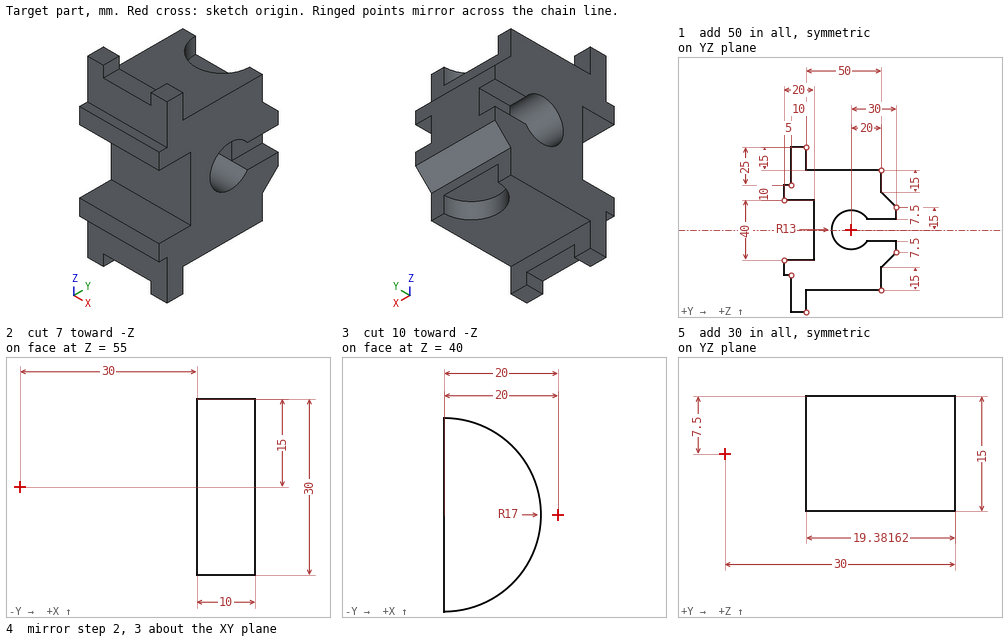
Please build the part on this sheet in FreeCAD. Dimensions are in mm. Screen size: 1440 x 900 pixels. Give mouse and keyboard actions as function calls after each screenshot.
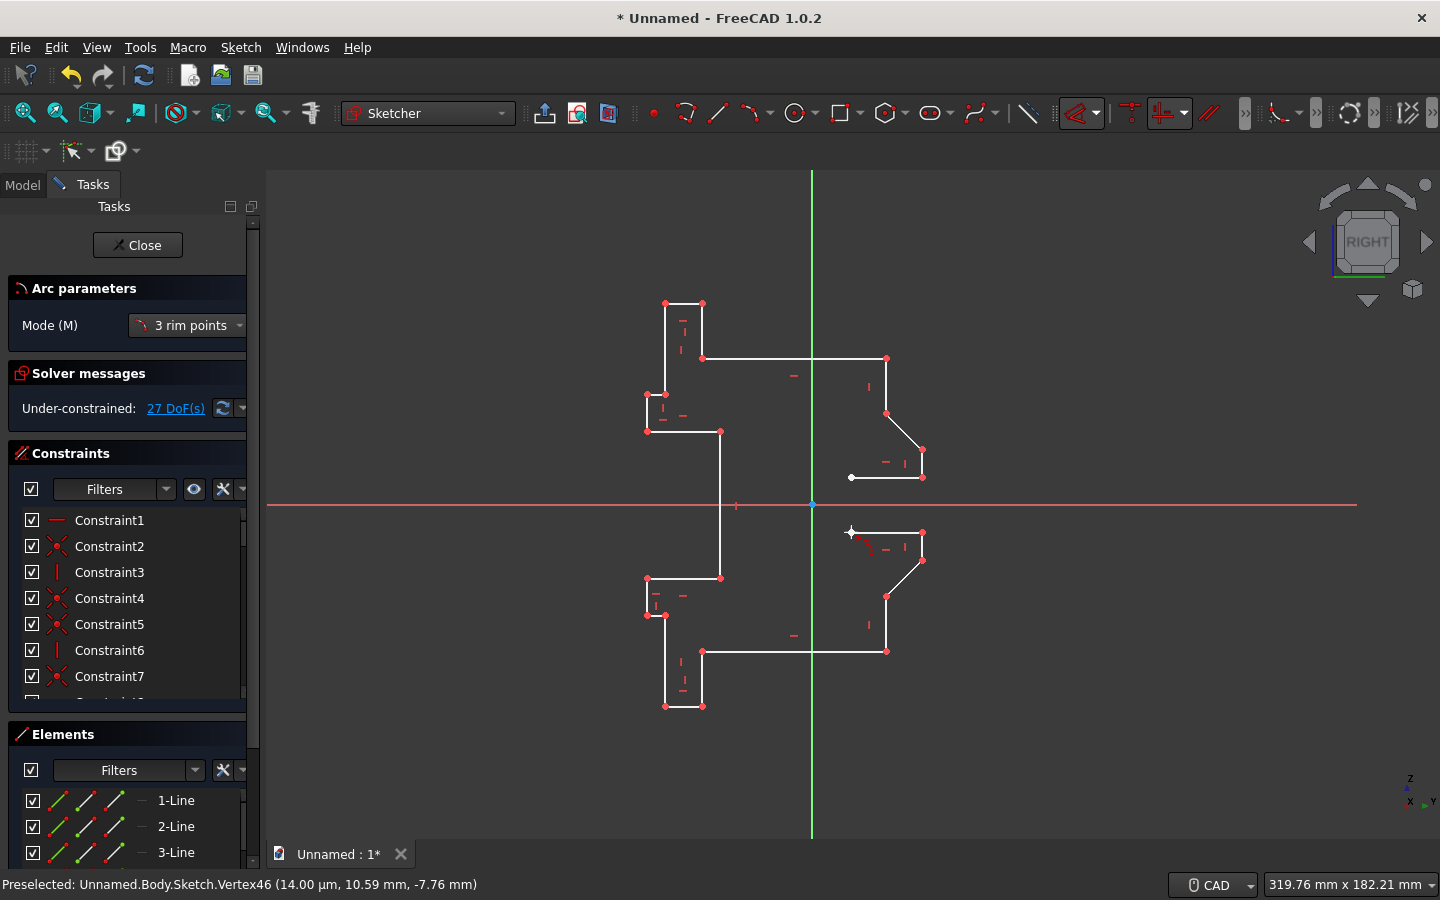
click(851, 533)
click(851, 478)
click(770, 481)
key(Escape)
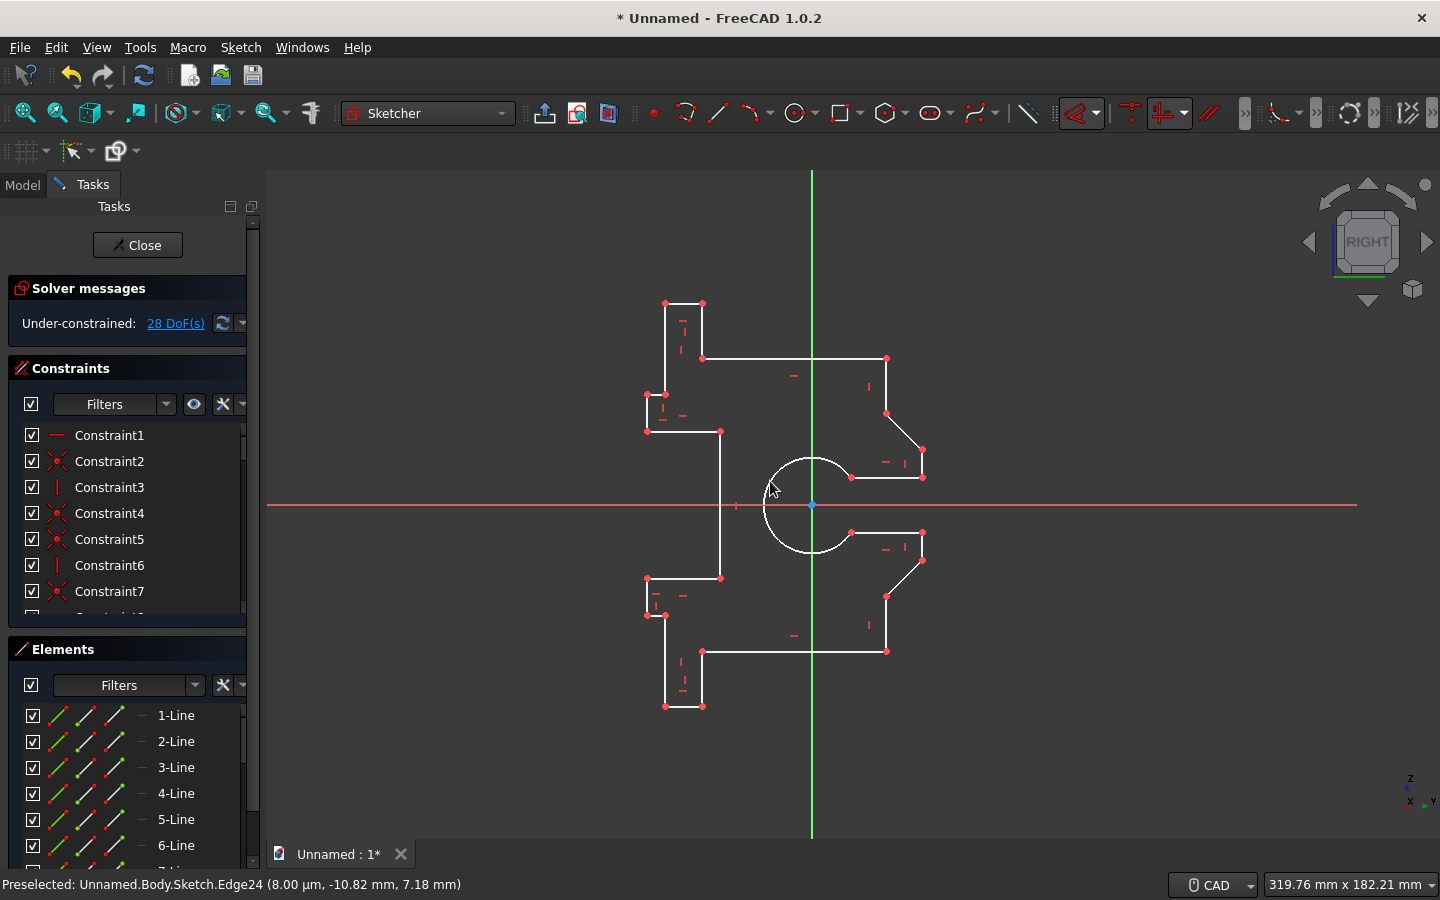
drag(802, 494, 822, 516)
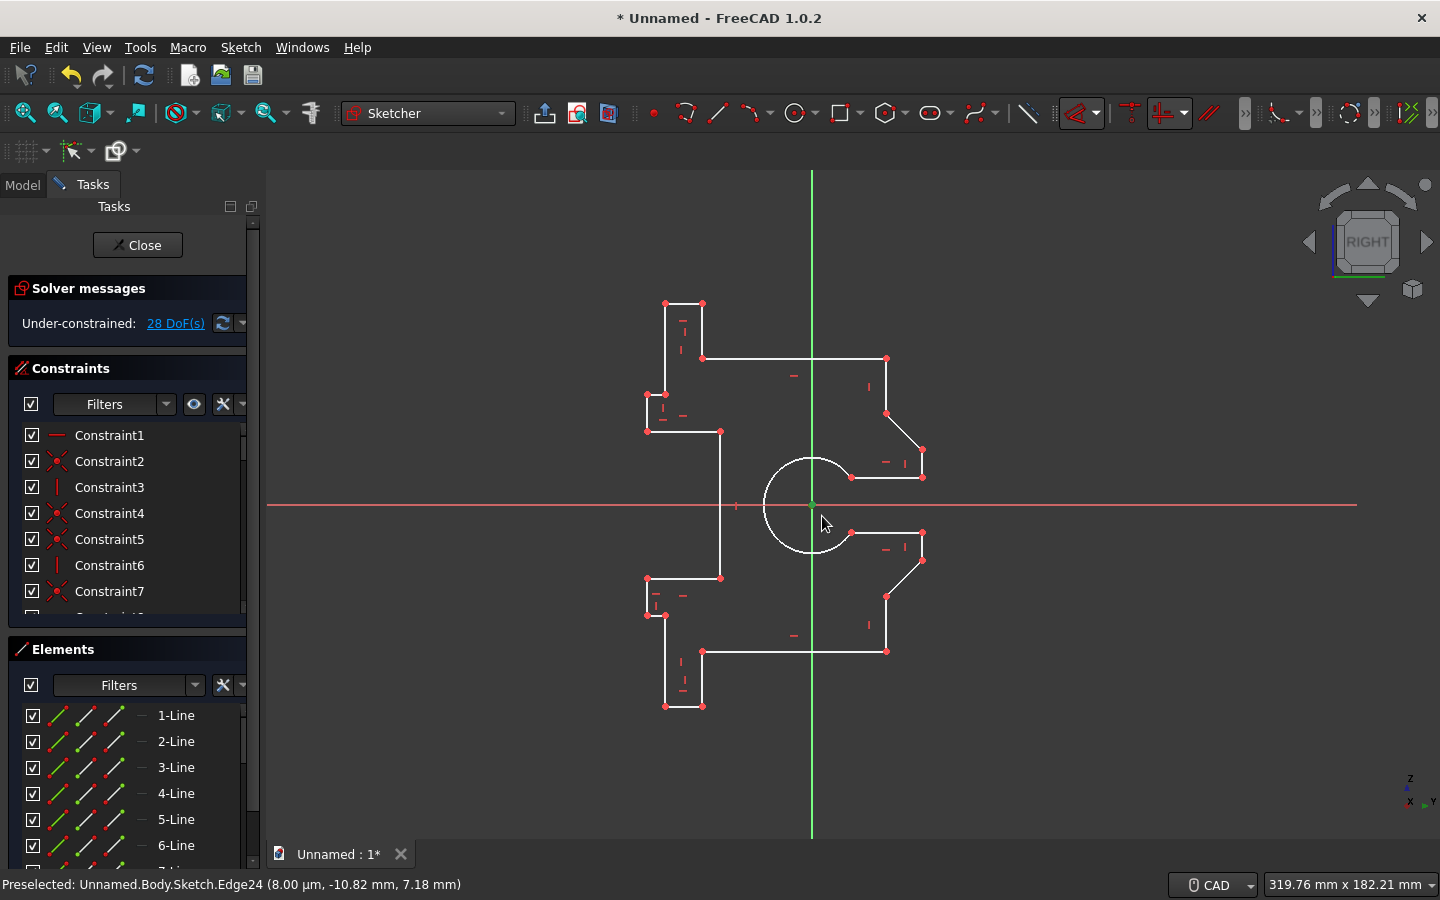
click(1130, 114)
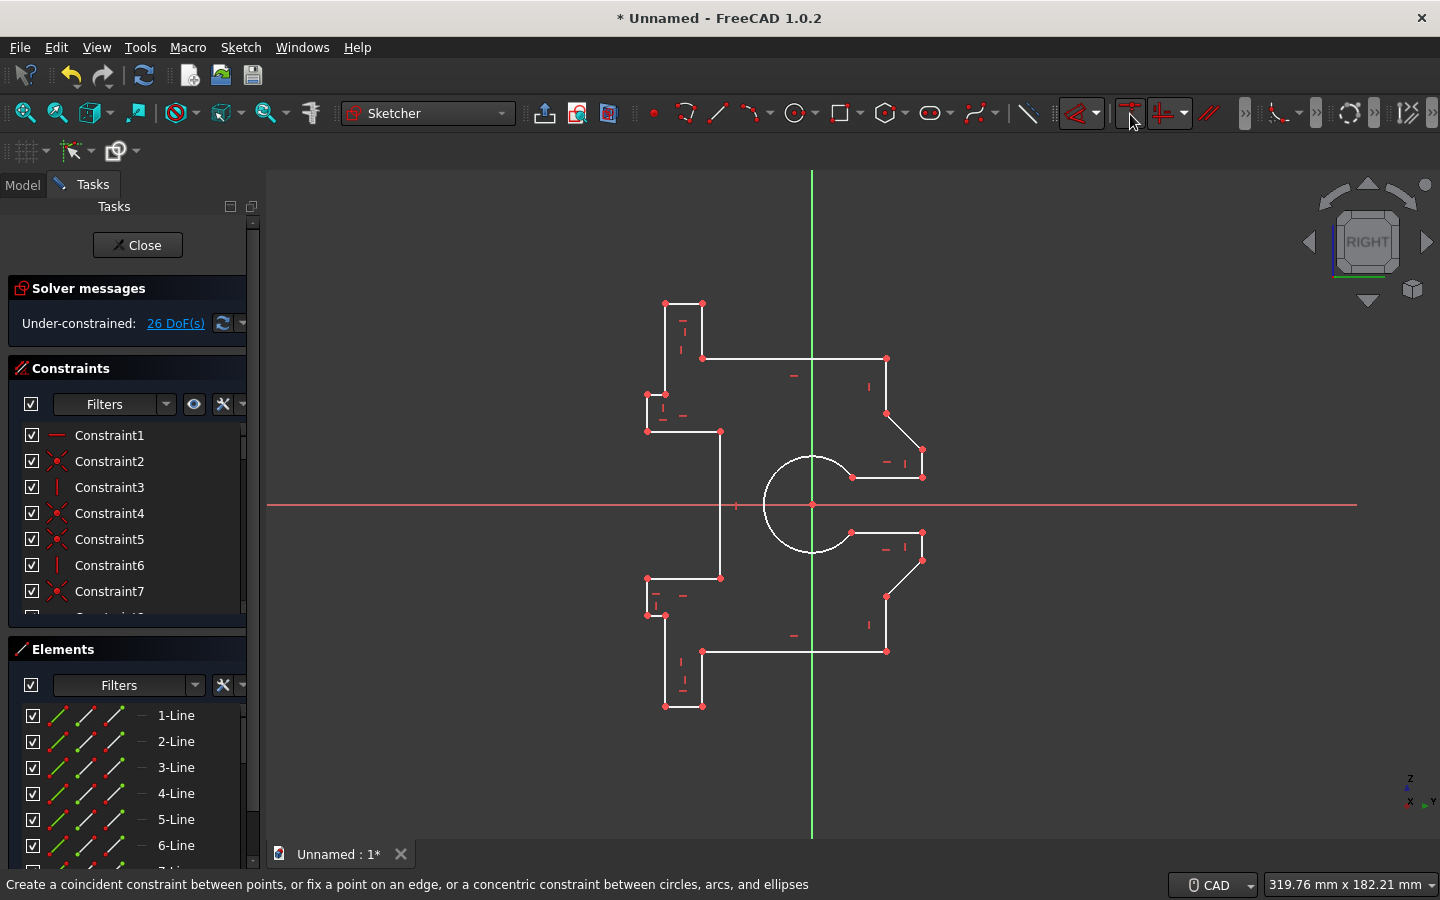
click(647, 432)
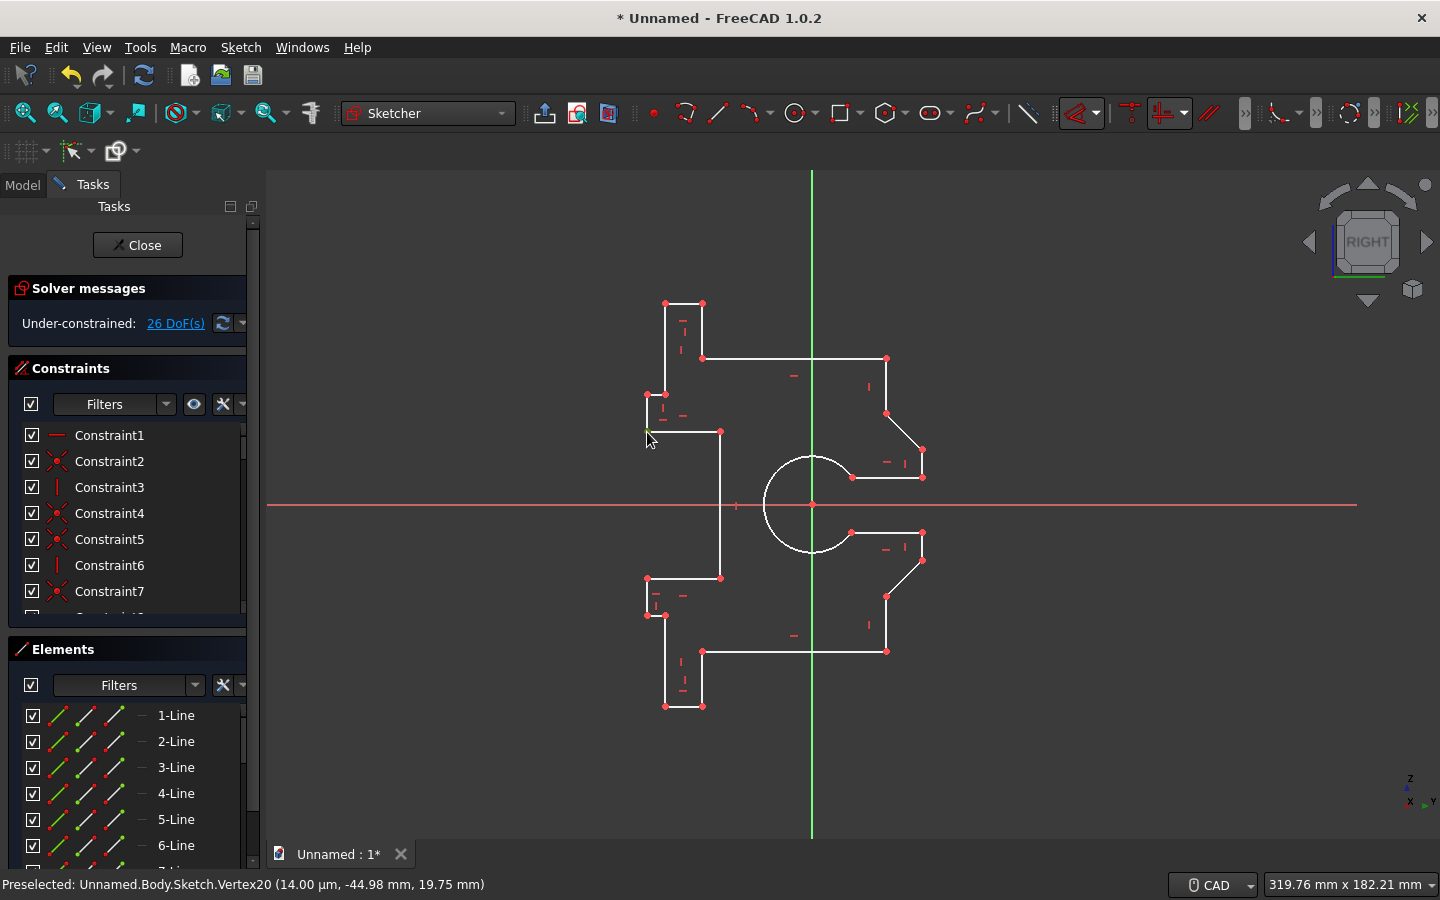
click(647, 579)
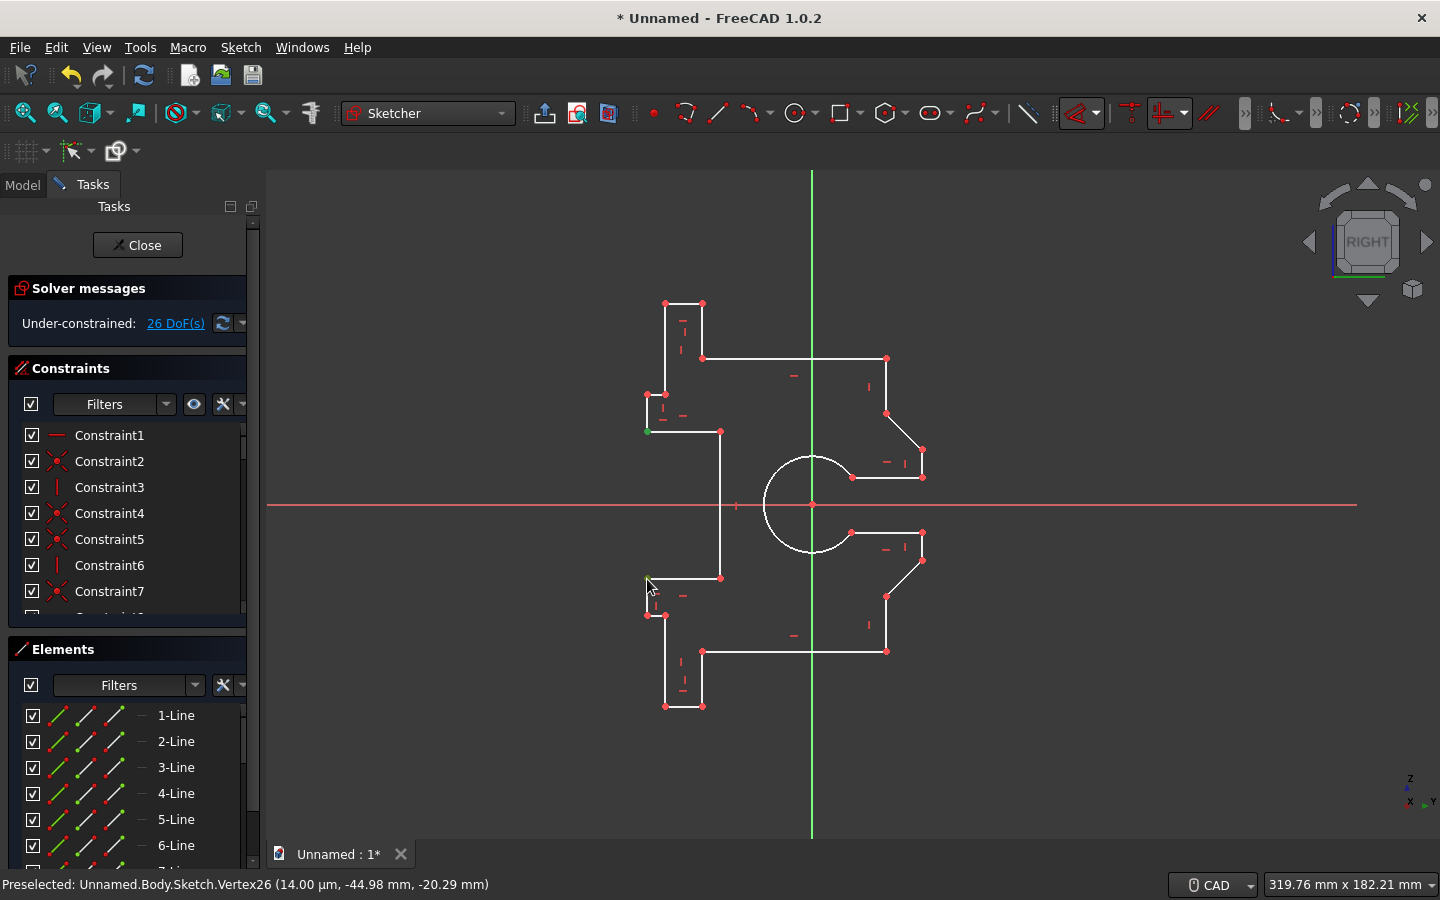
click(364, 504)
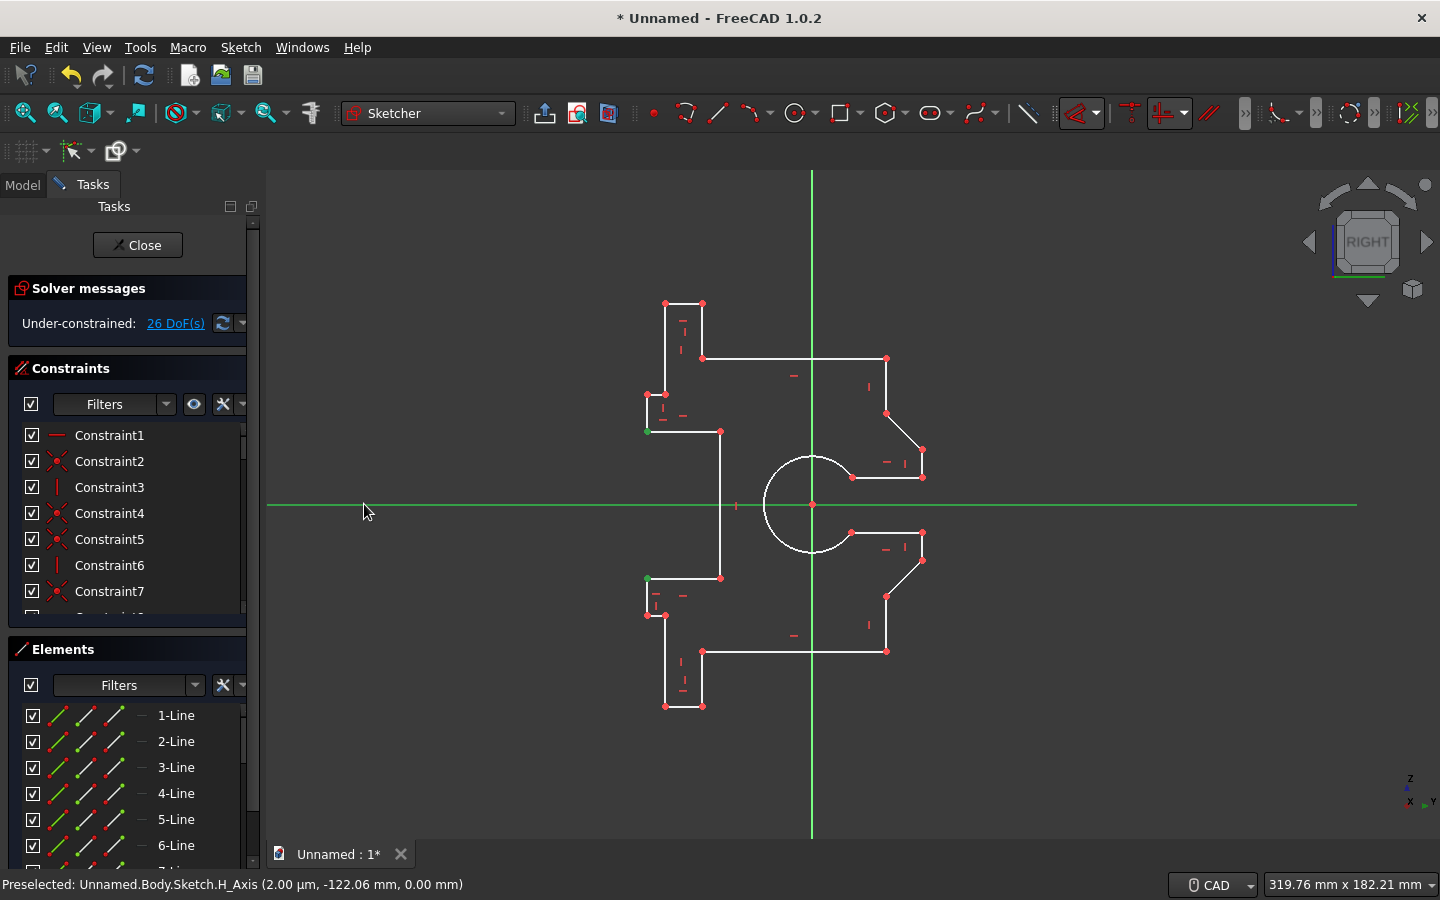
key(s)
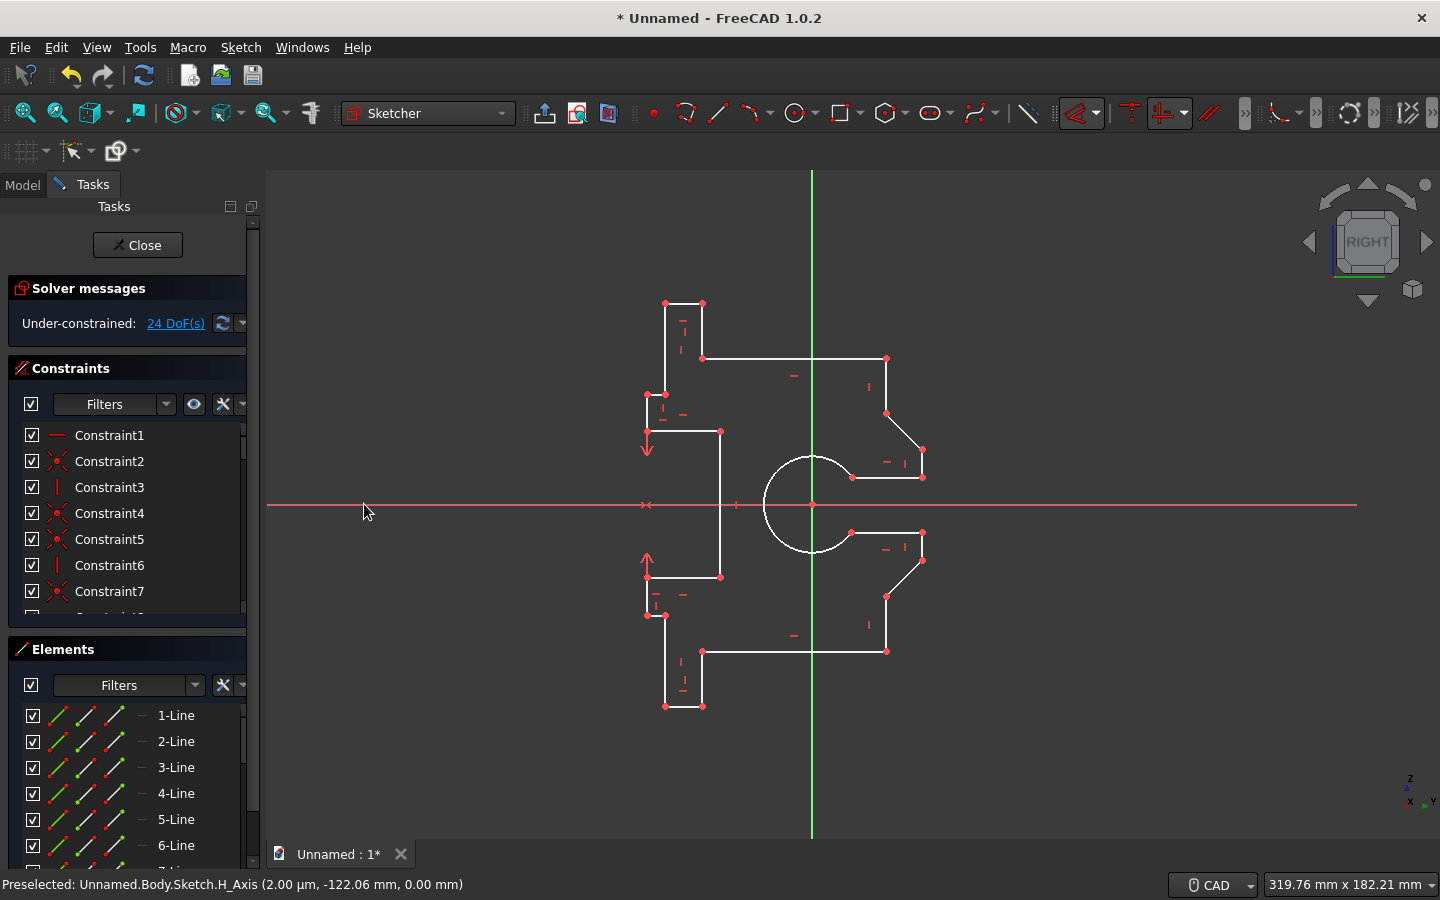
click(665, 395)